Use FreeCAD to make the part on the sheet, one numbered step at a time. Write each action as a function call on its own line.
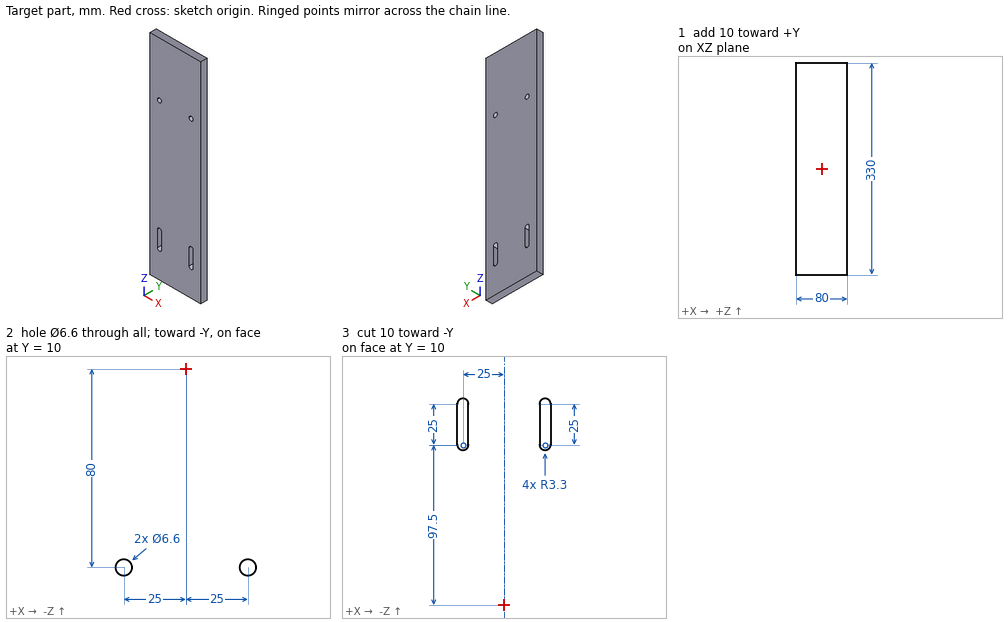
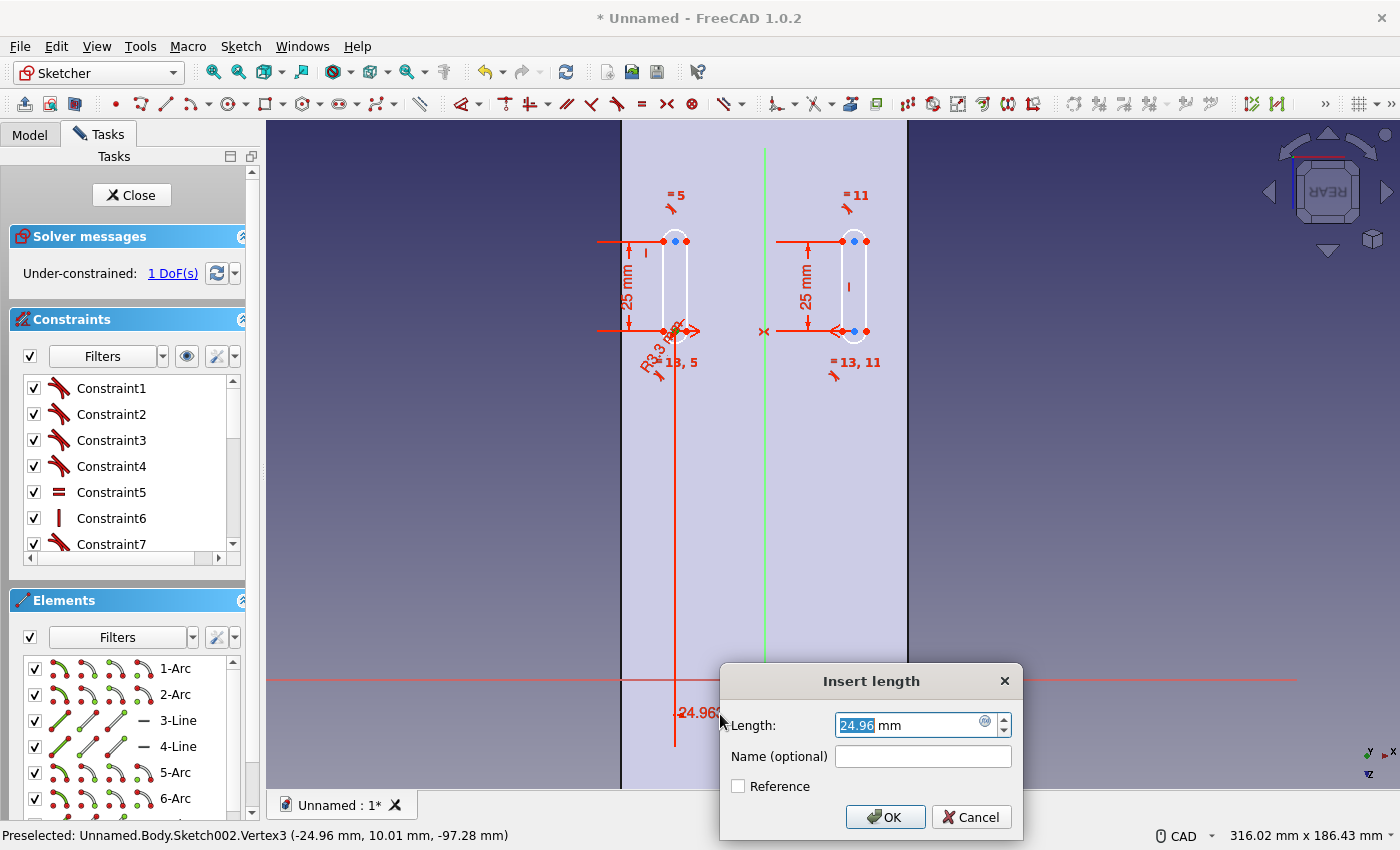
text(25)
key(Return)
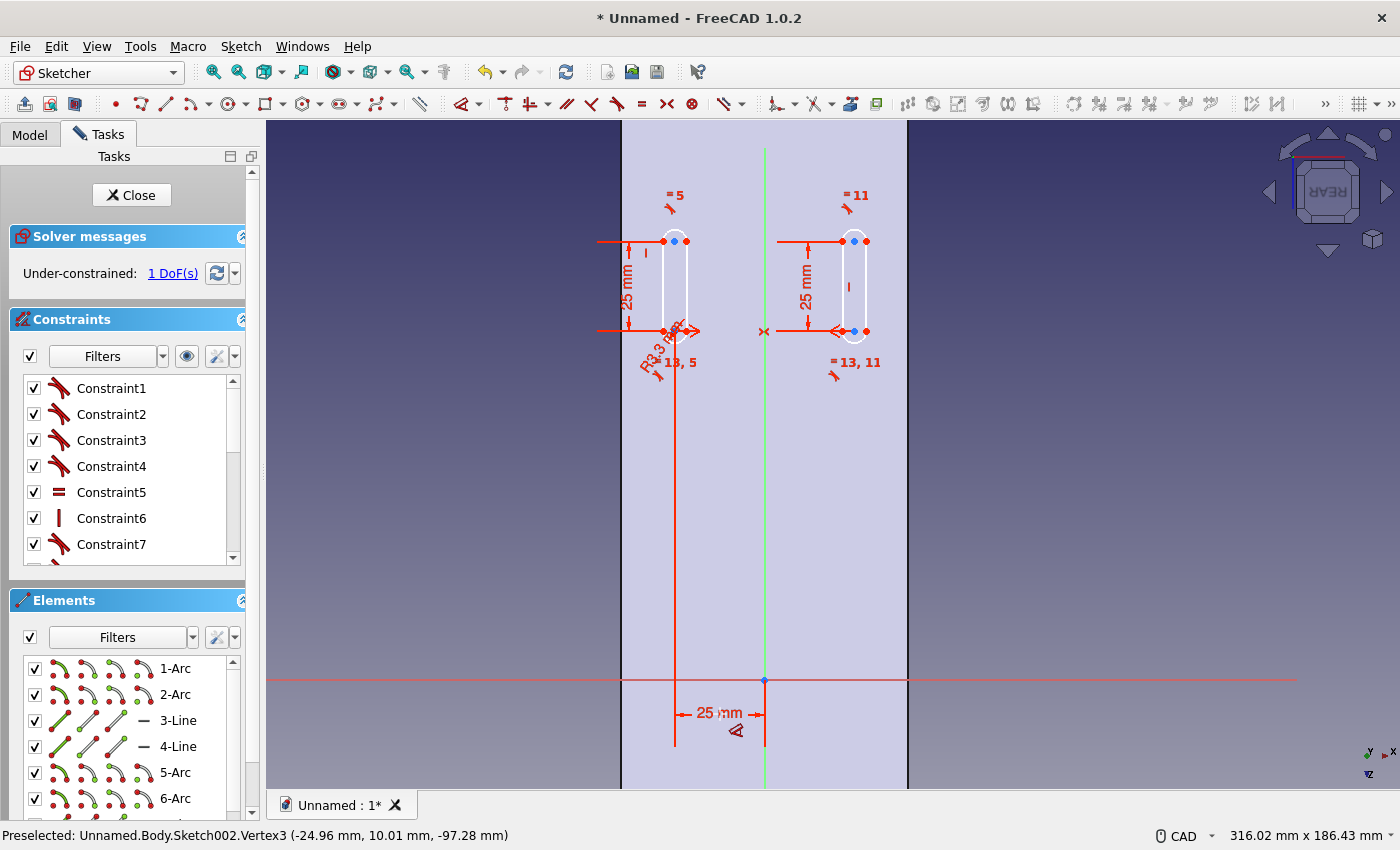
click(663, 331)
click(629, 506)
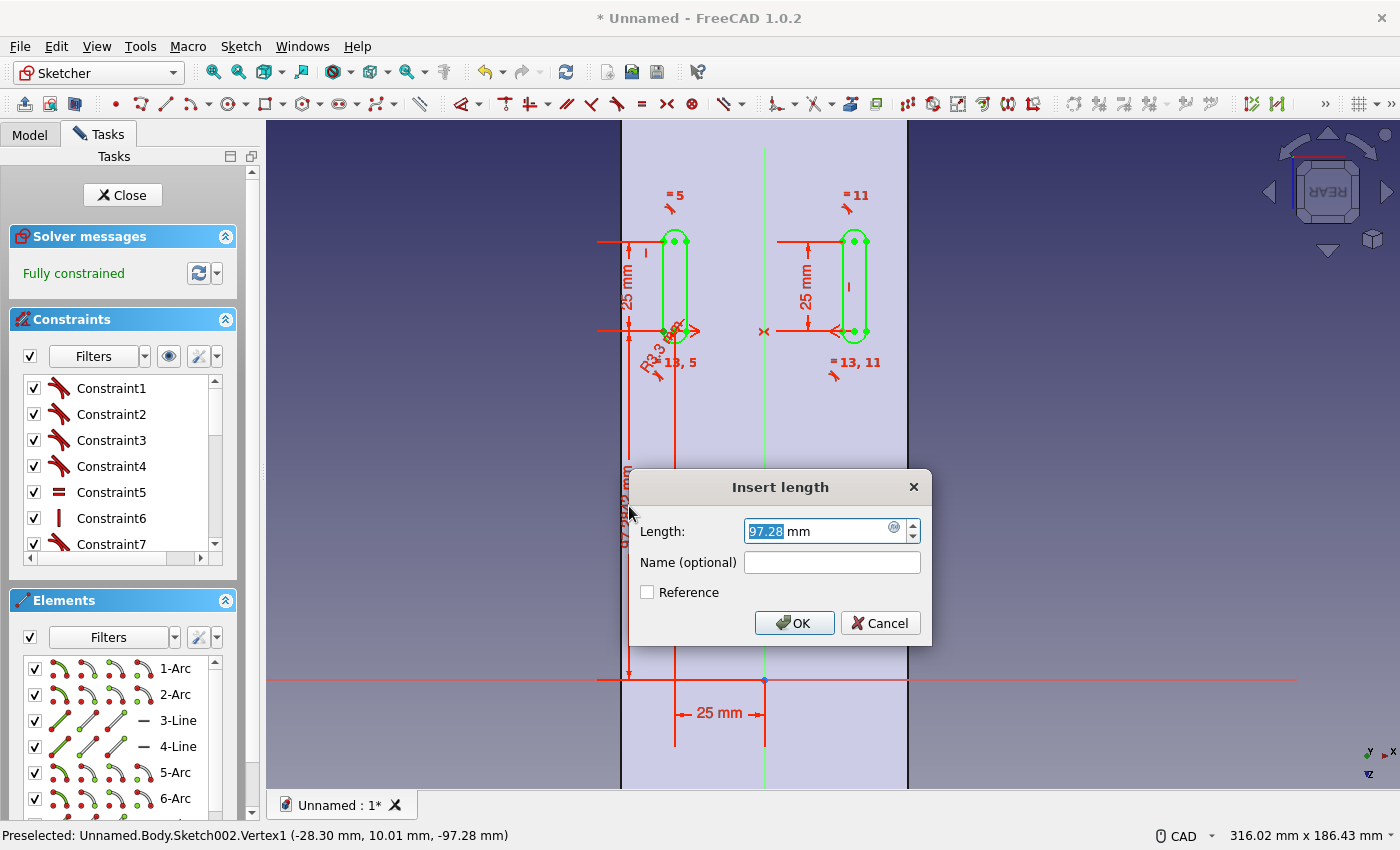
text(97.5)
key(Return)
key(Escape)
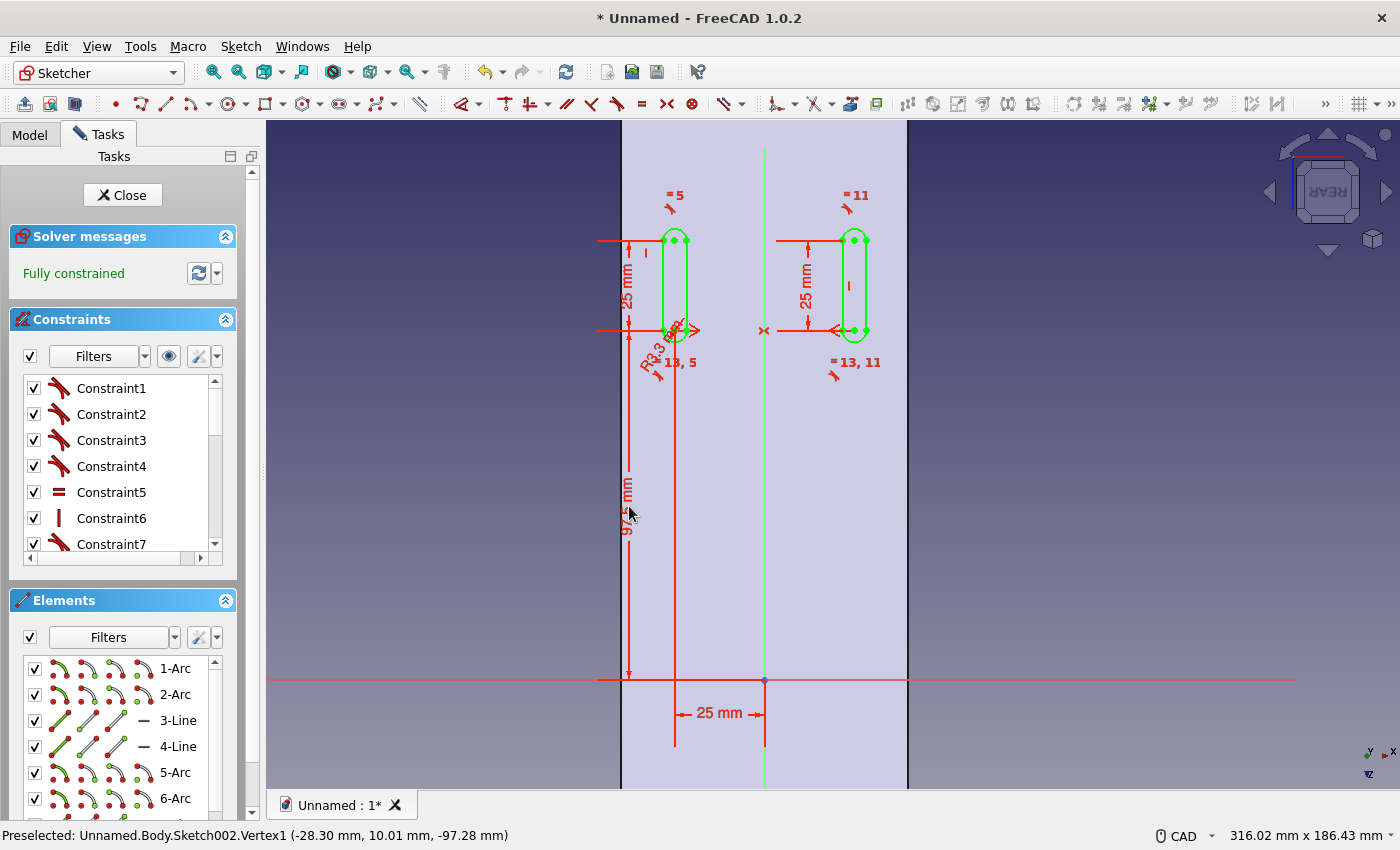
click(123, 195)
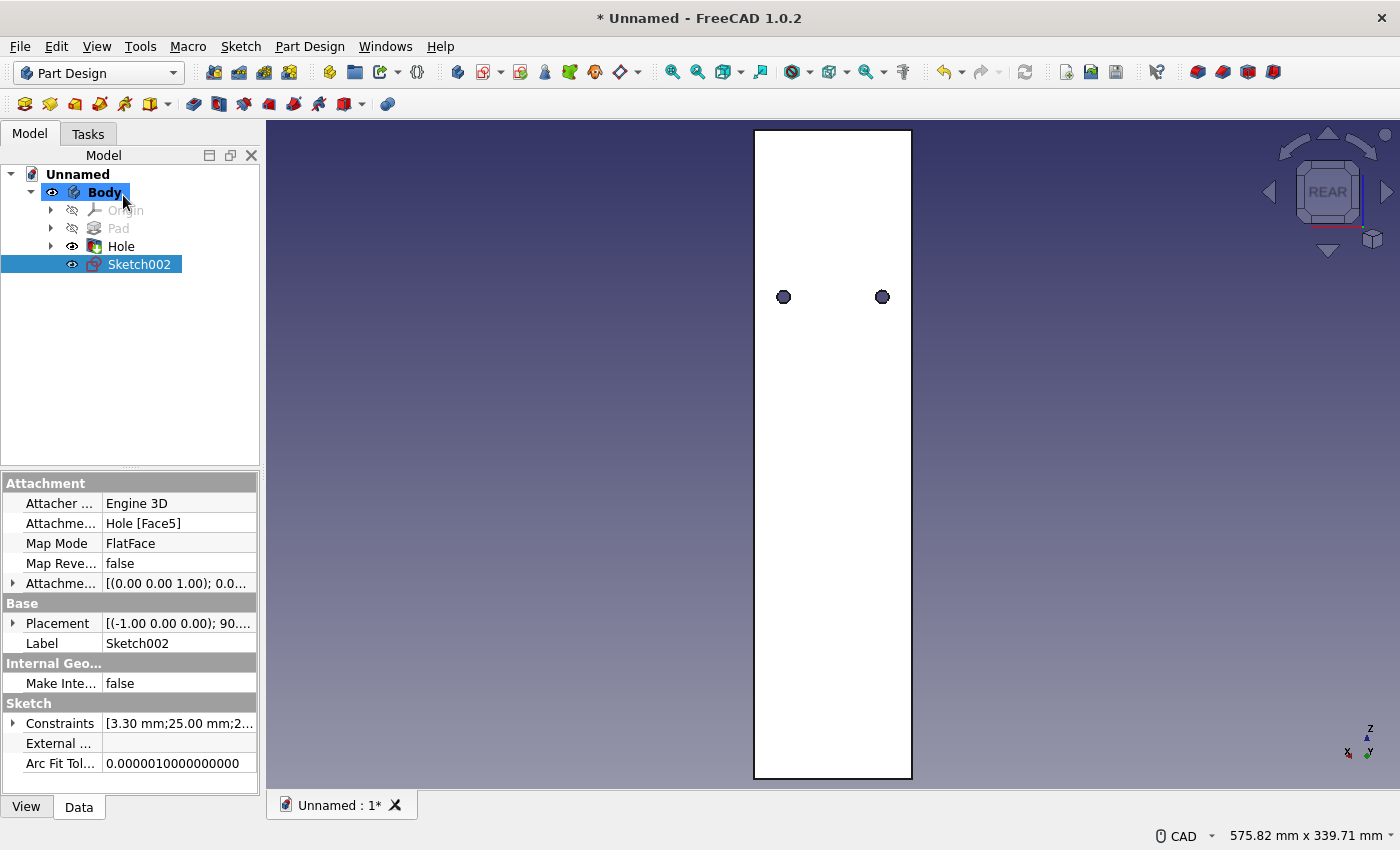
click(194, 104)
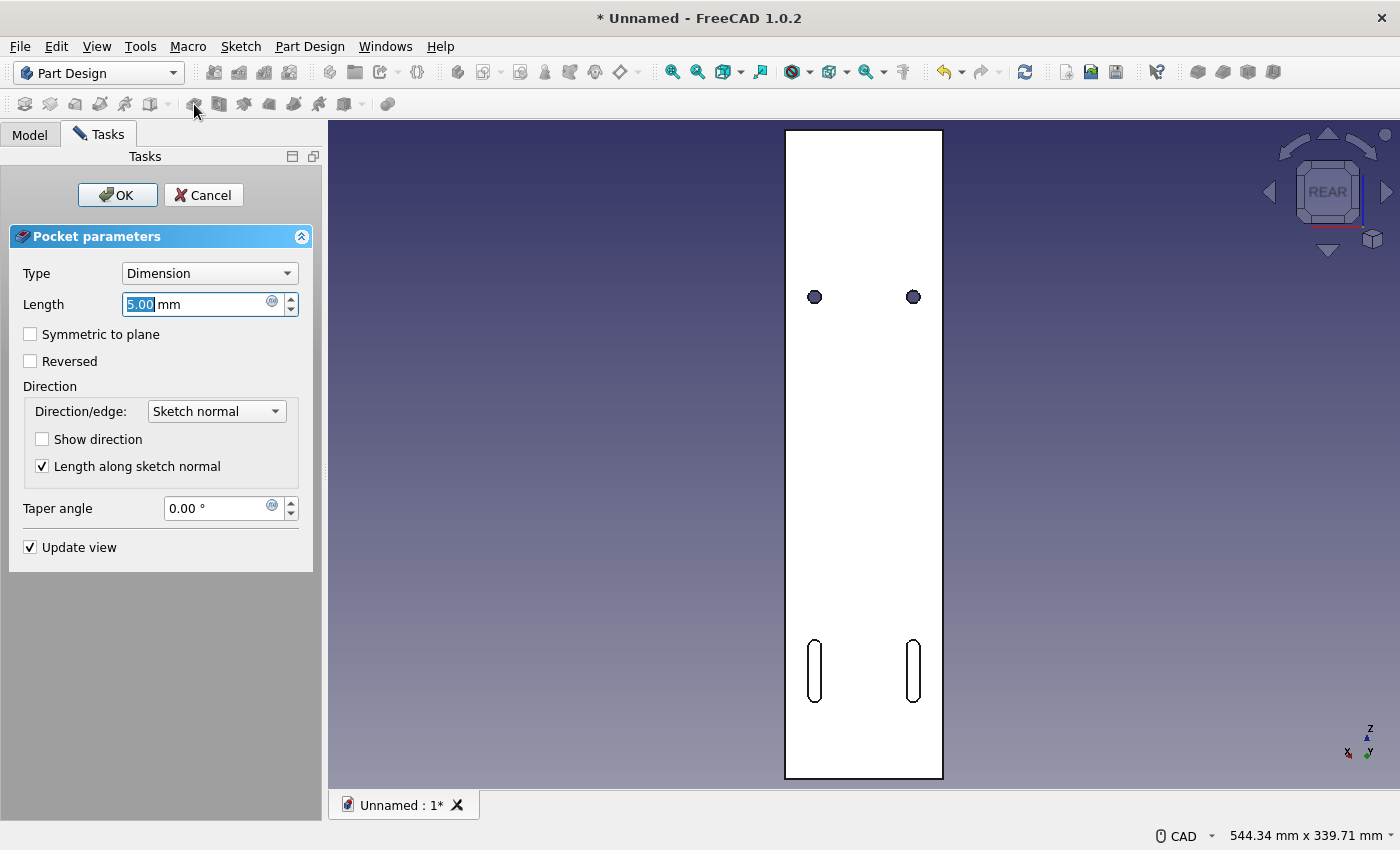
text(10)
key(Tab)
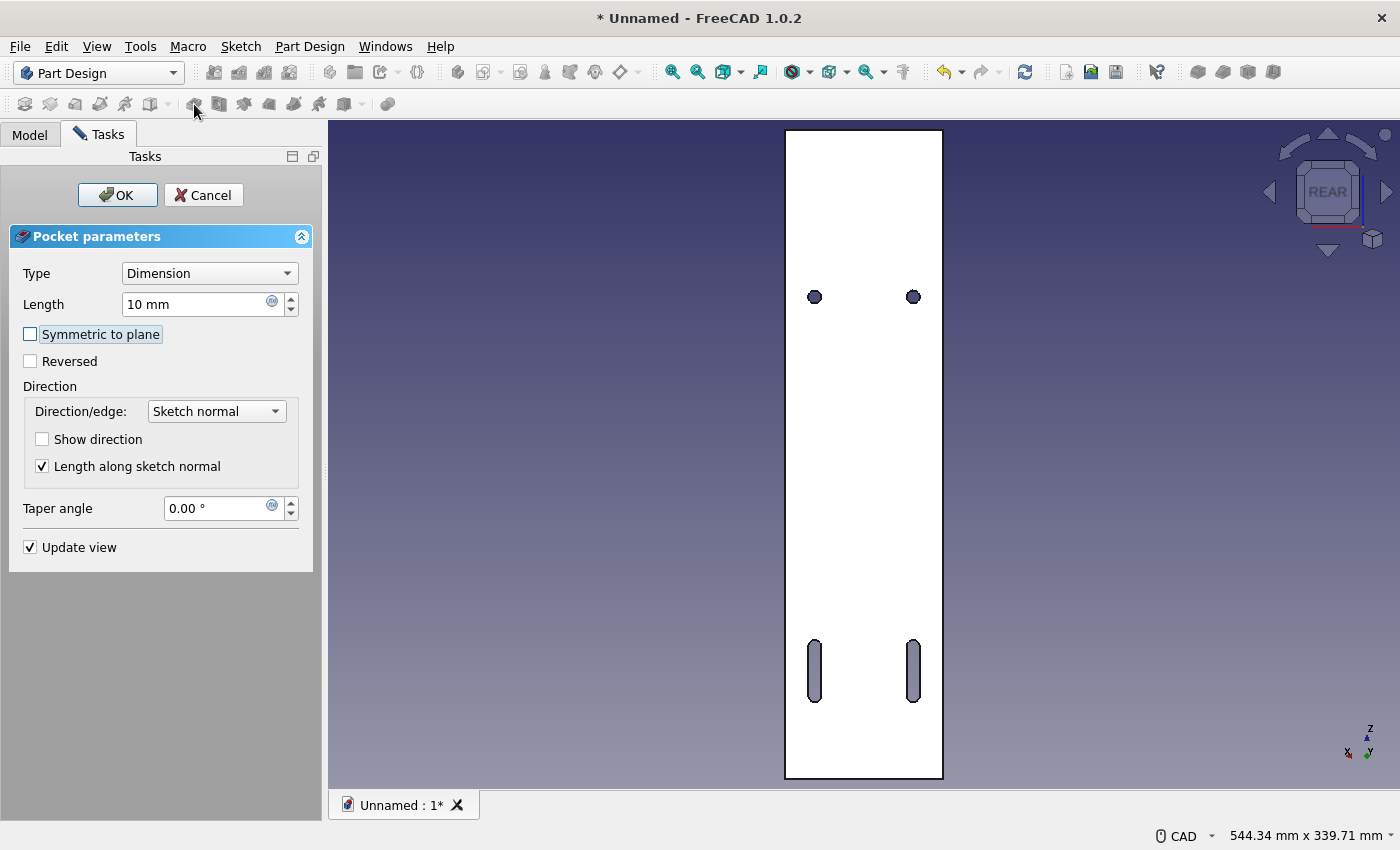
click(118, 195)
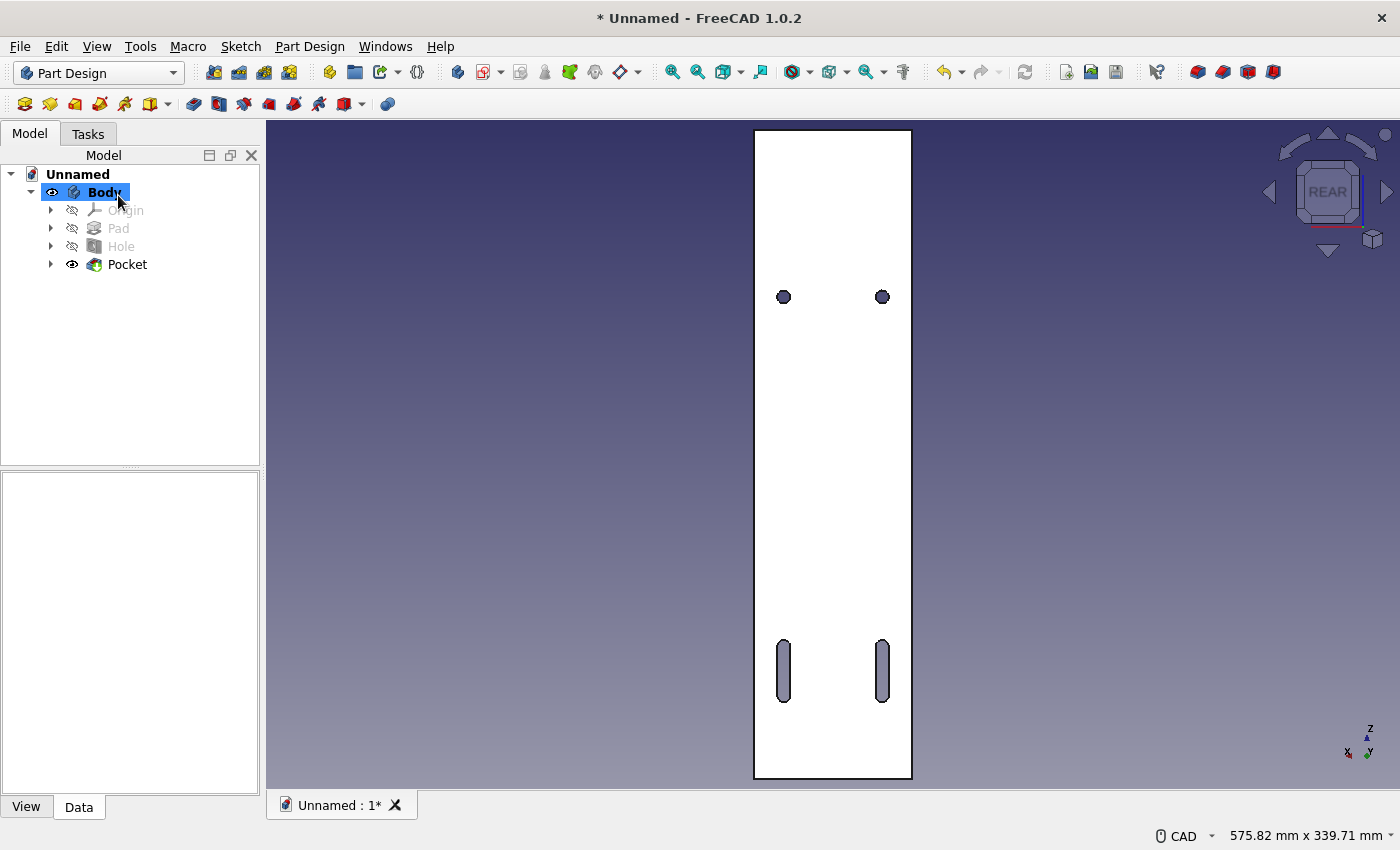
key(0)